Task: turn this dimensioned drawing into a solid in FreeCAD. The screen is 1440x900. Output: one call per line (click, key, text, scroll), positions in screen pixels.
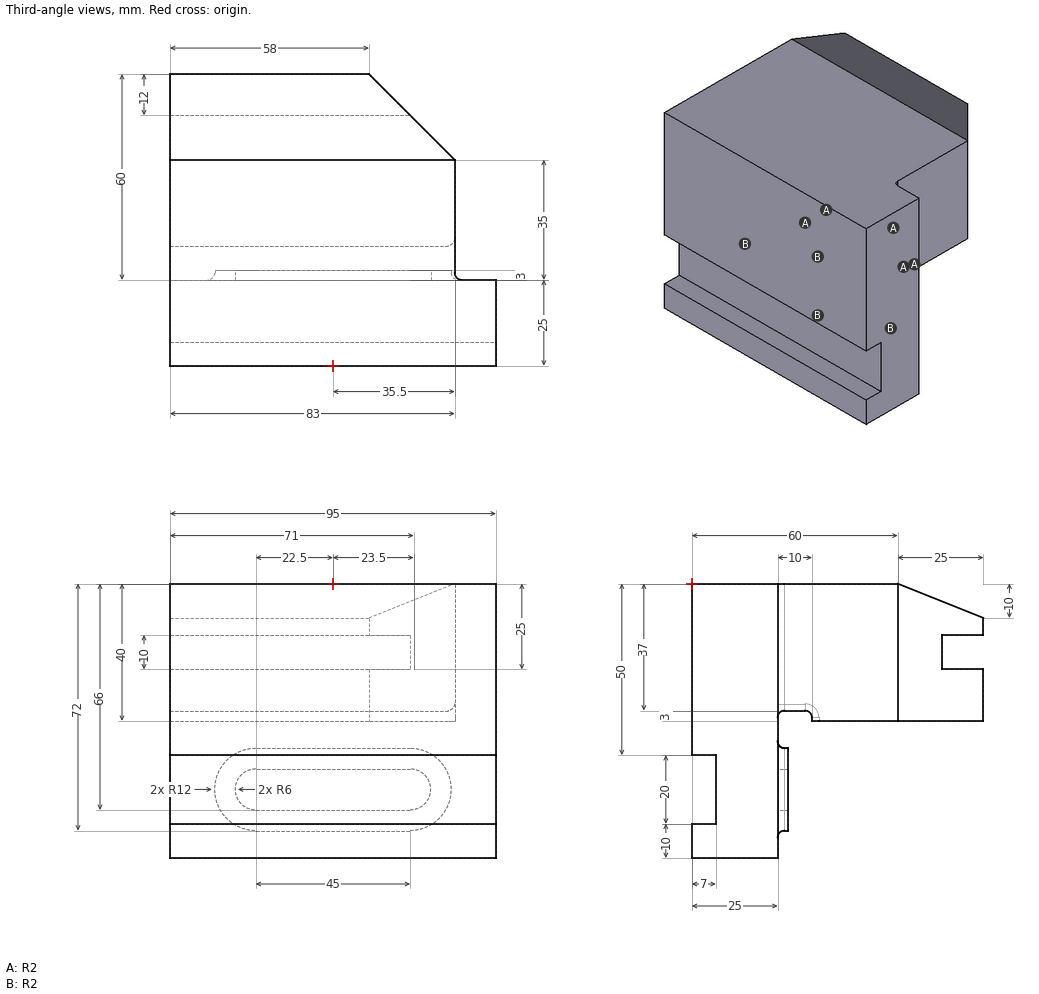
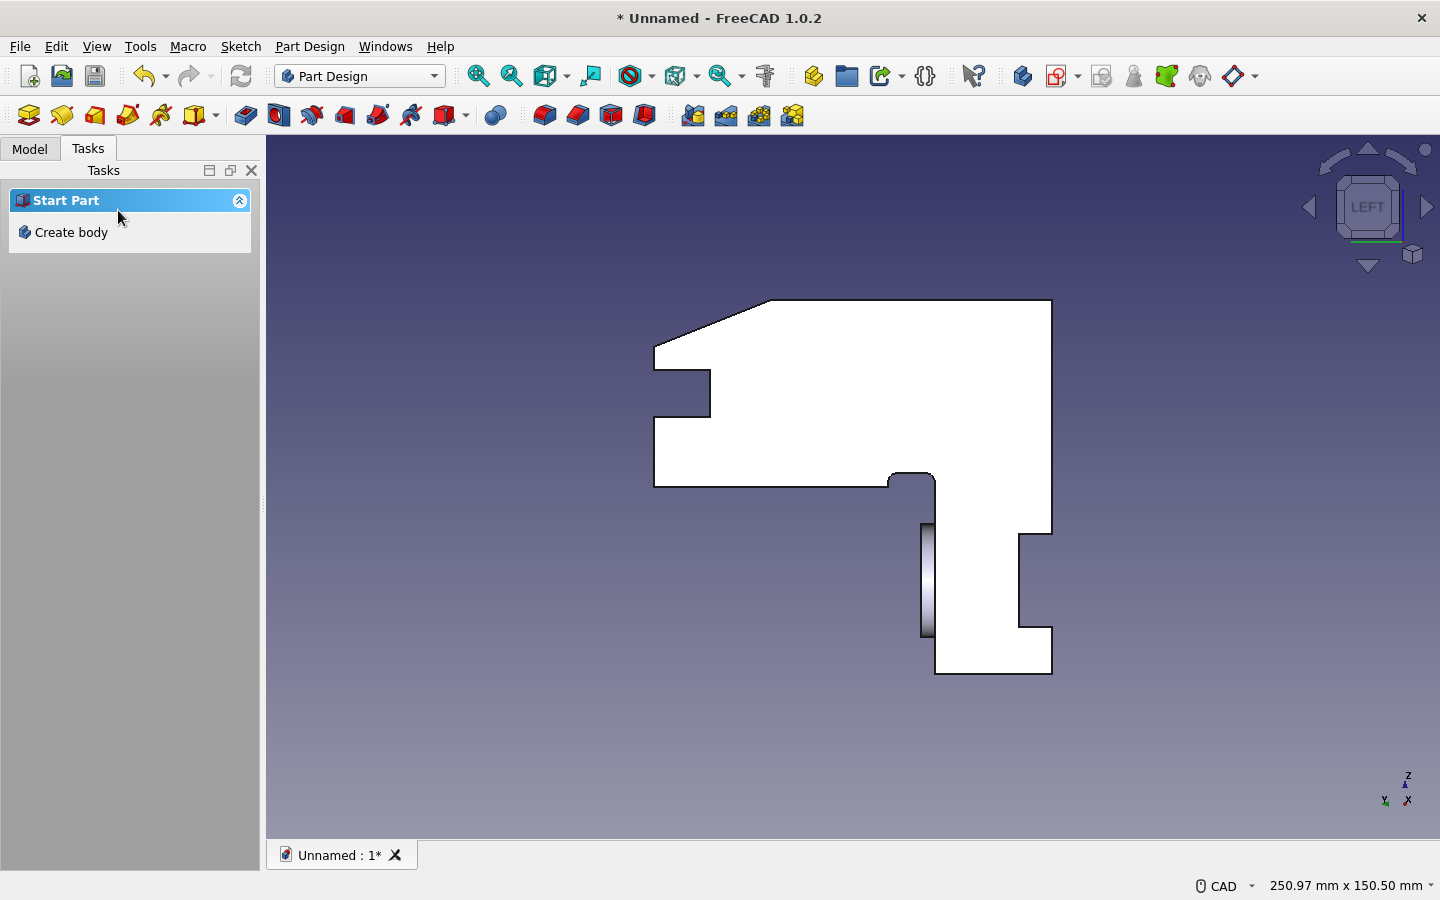
key(v)
key(3)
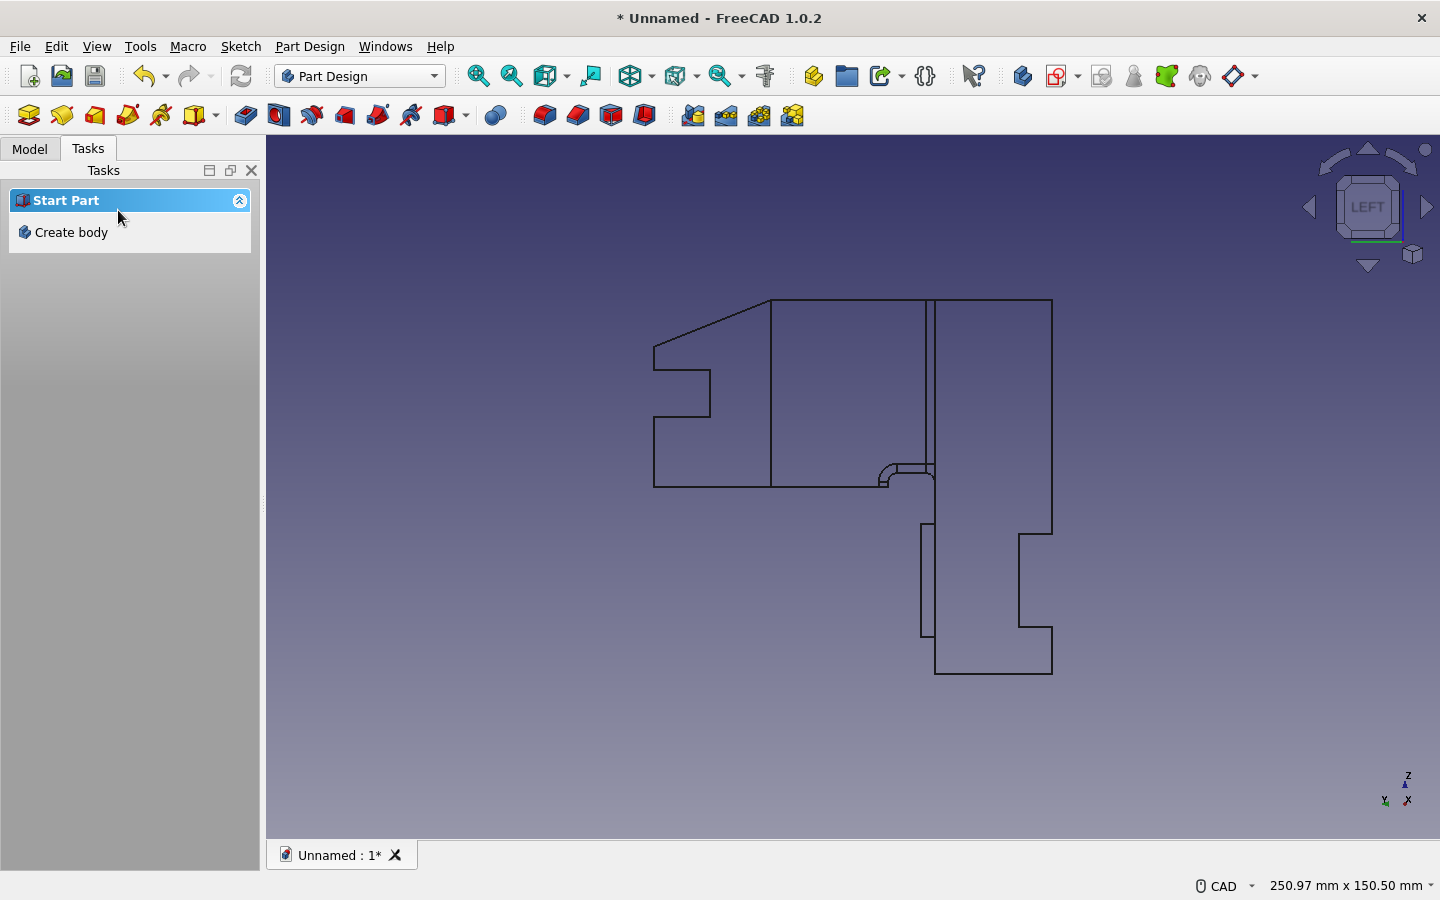
key(0)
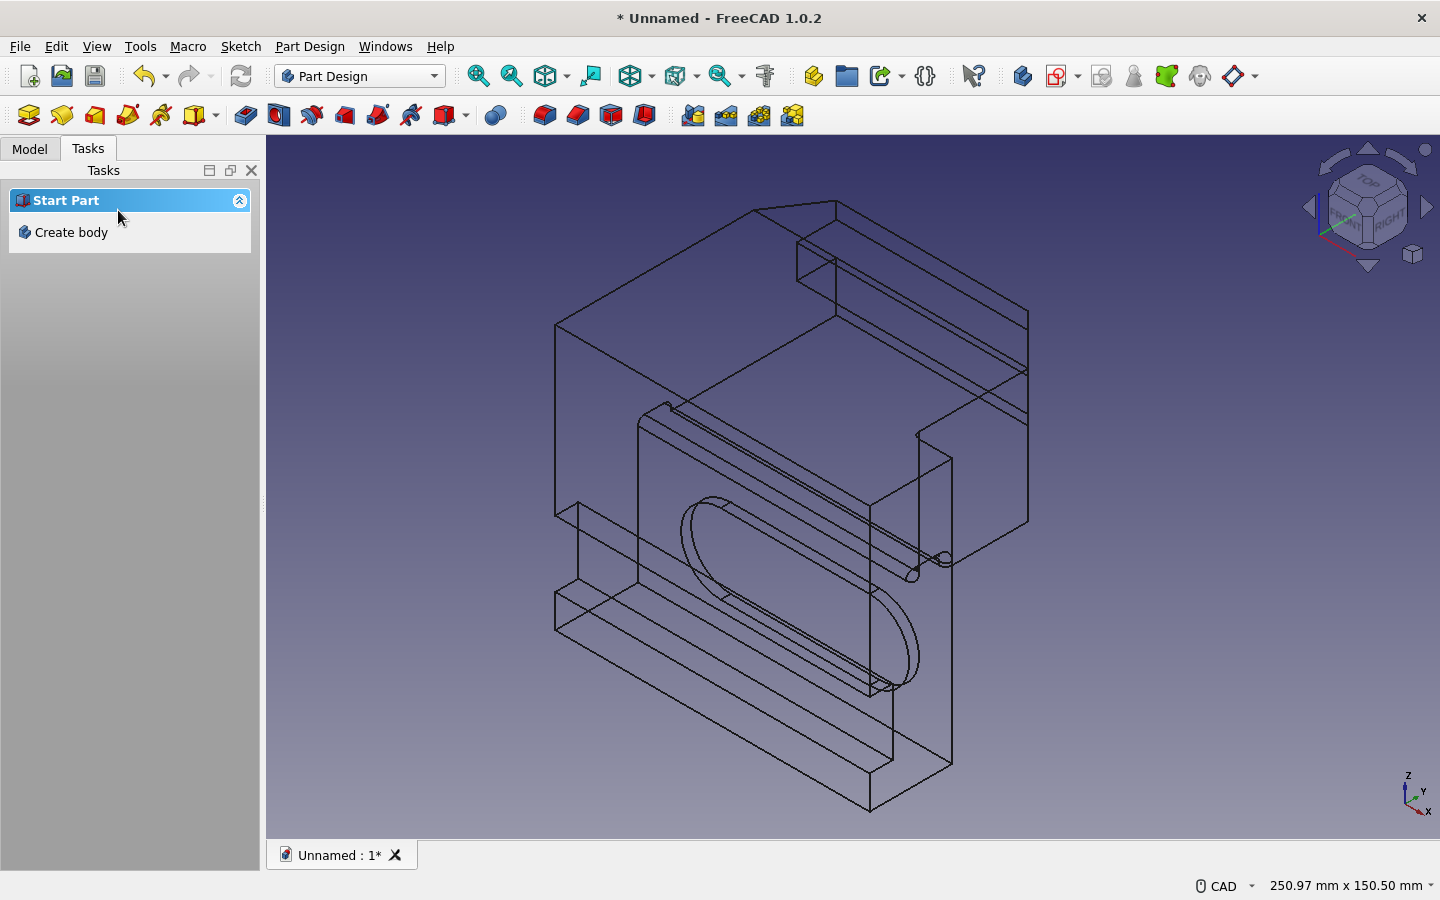
click(681, 530)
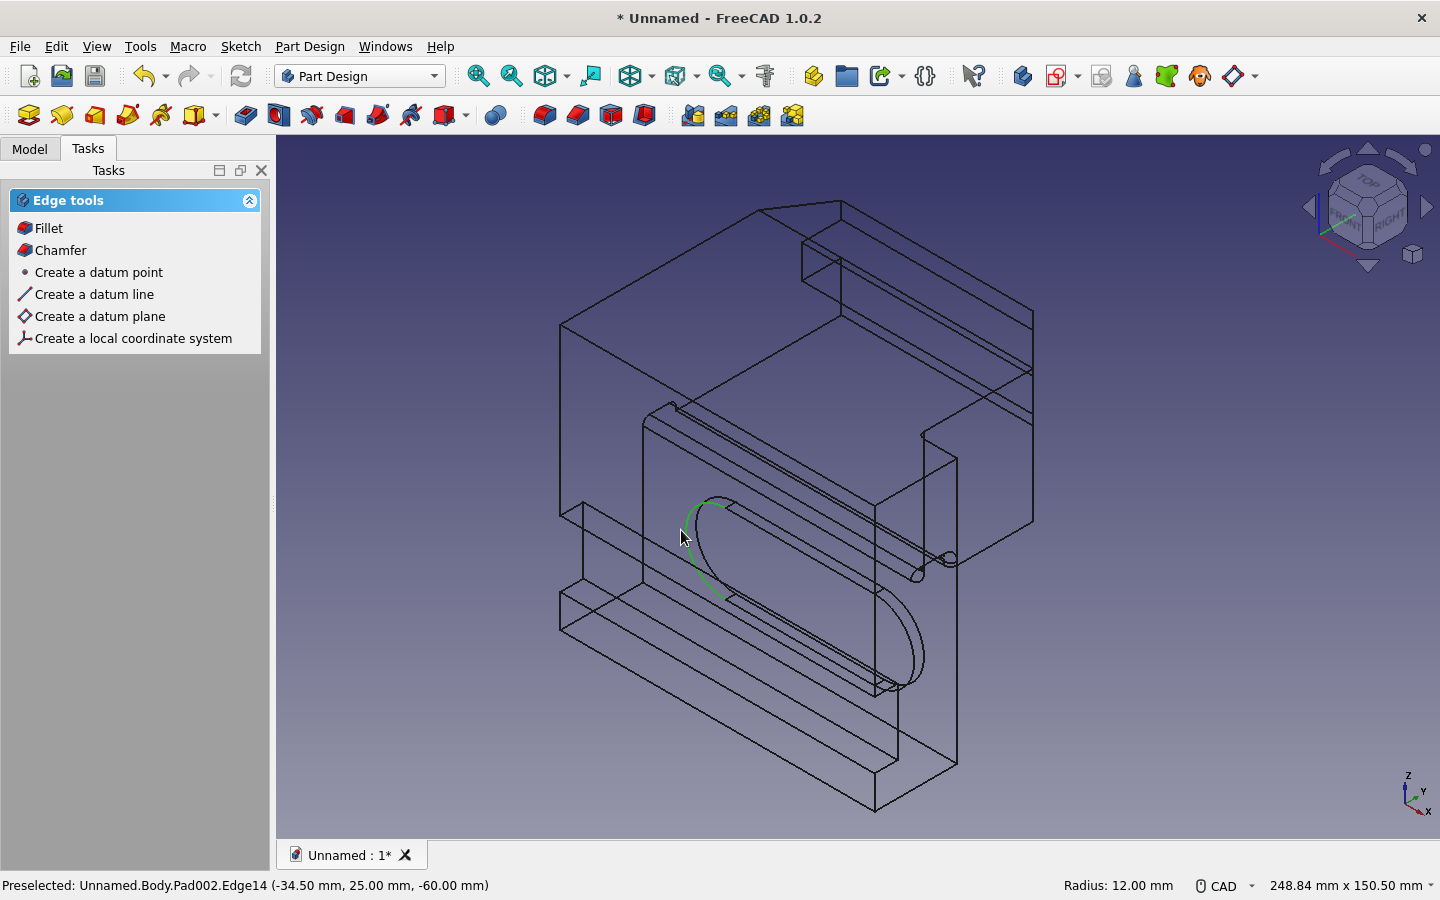
click(800, 550, ctrl)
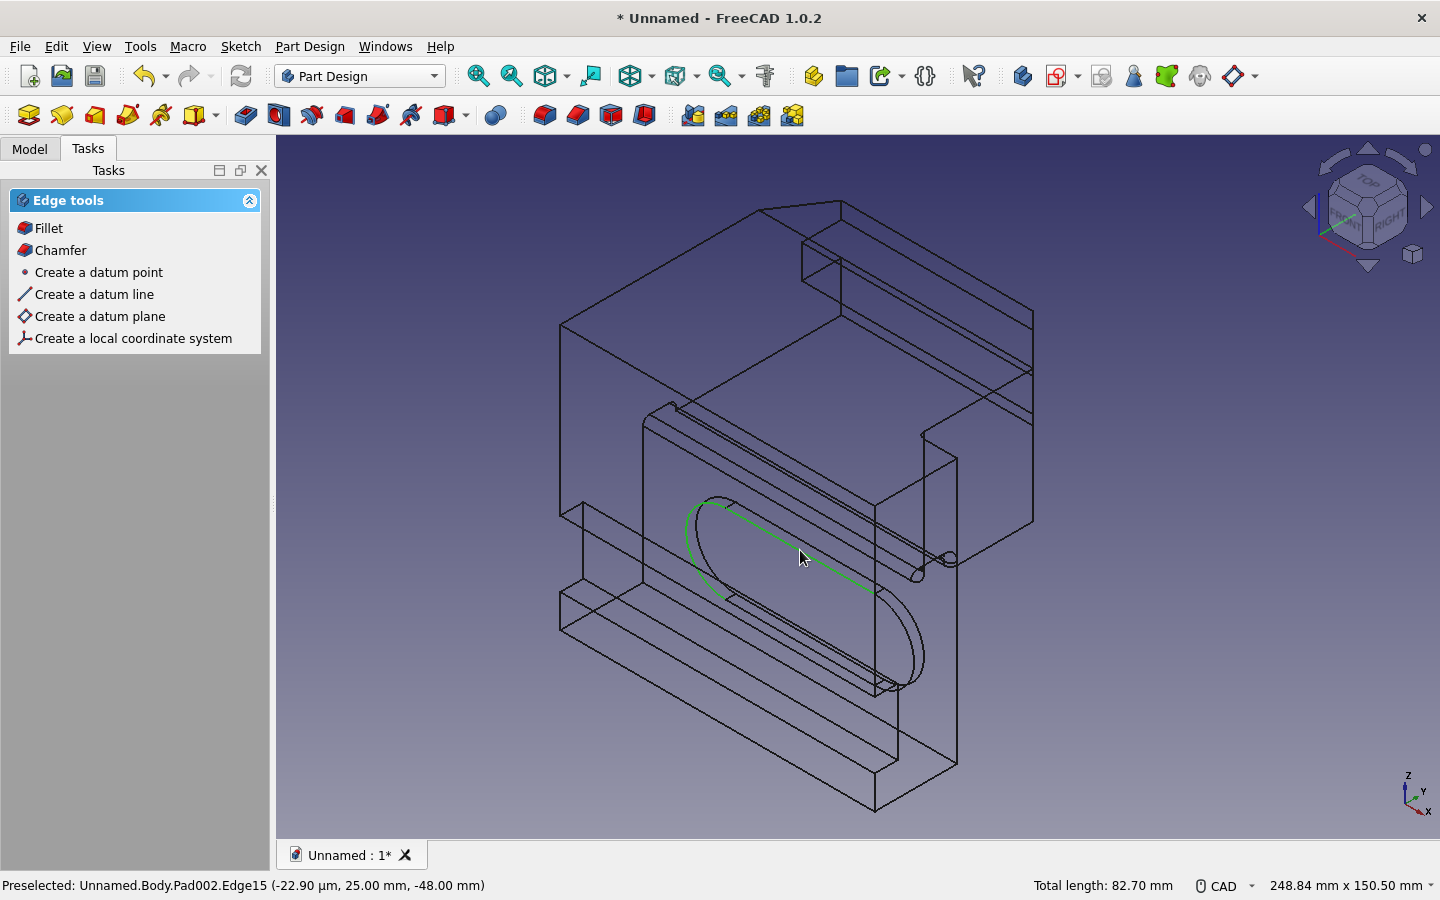
click(914, 662, ctrl)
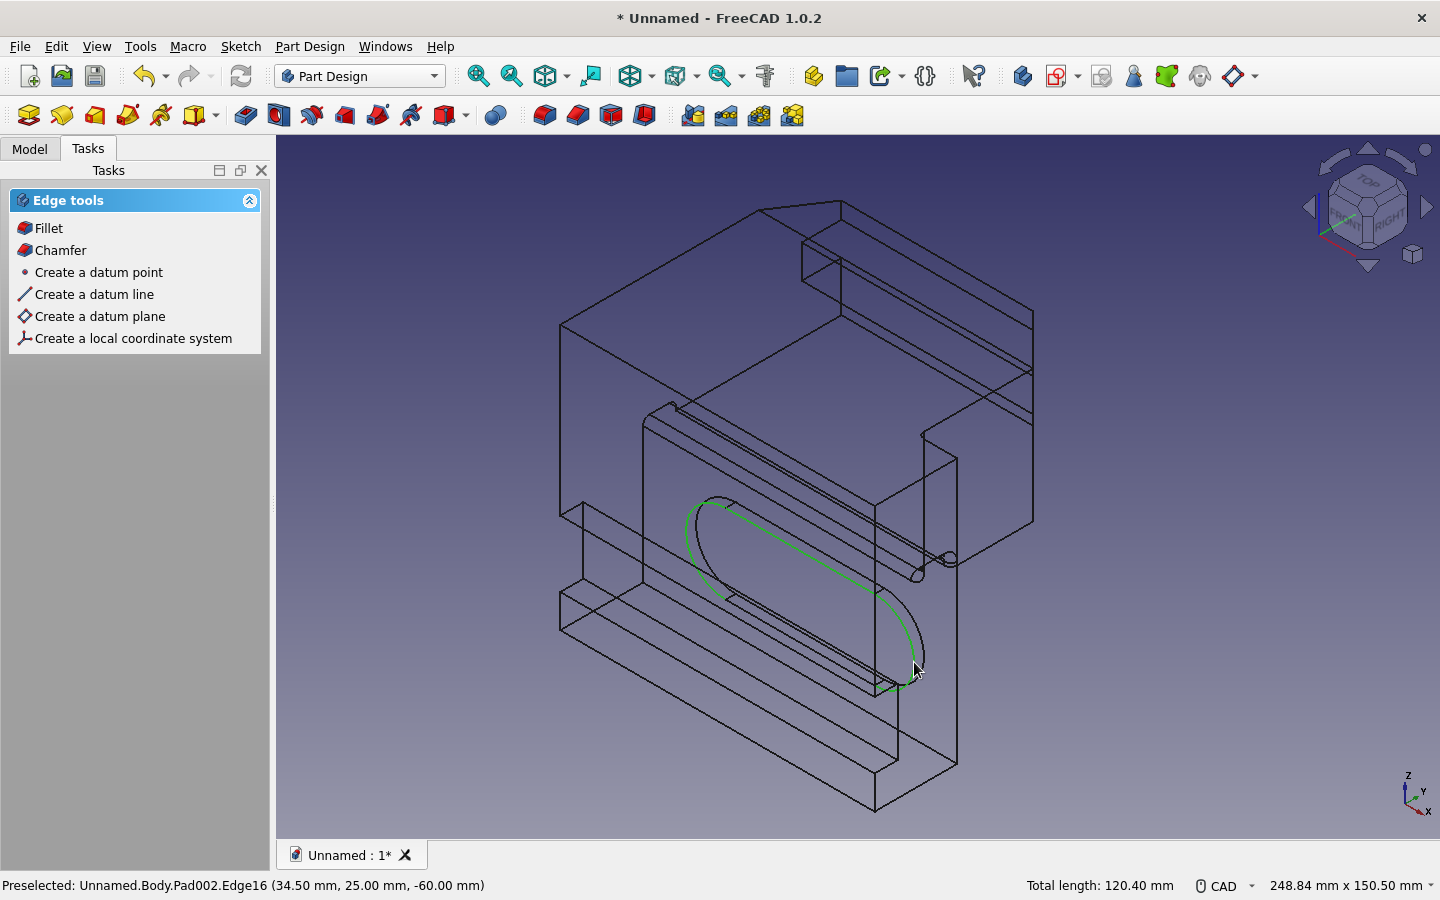
click(800, 642, ctrl)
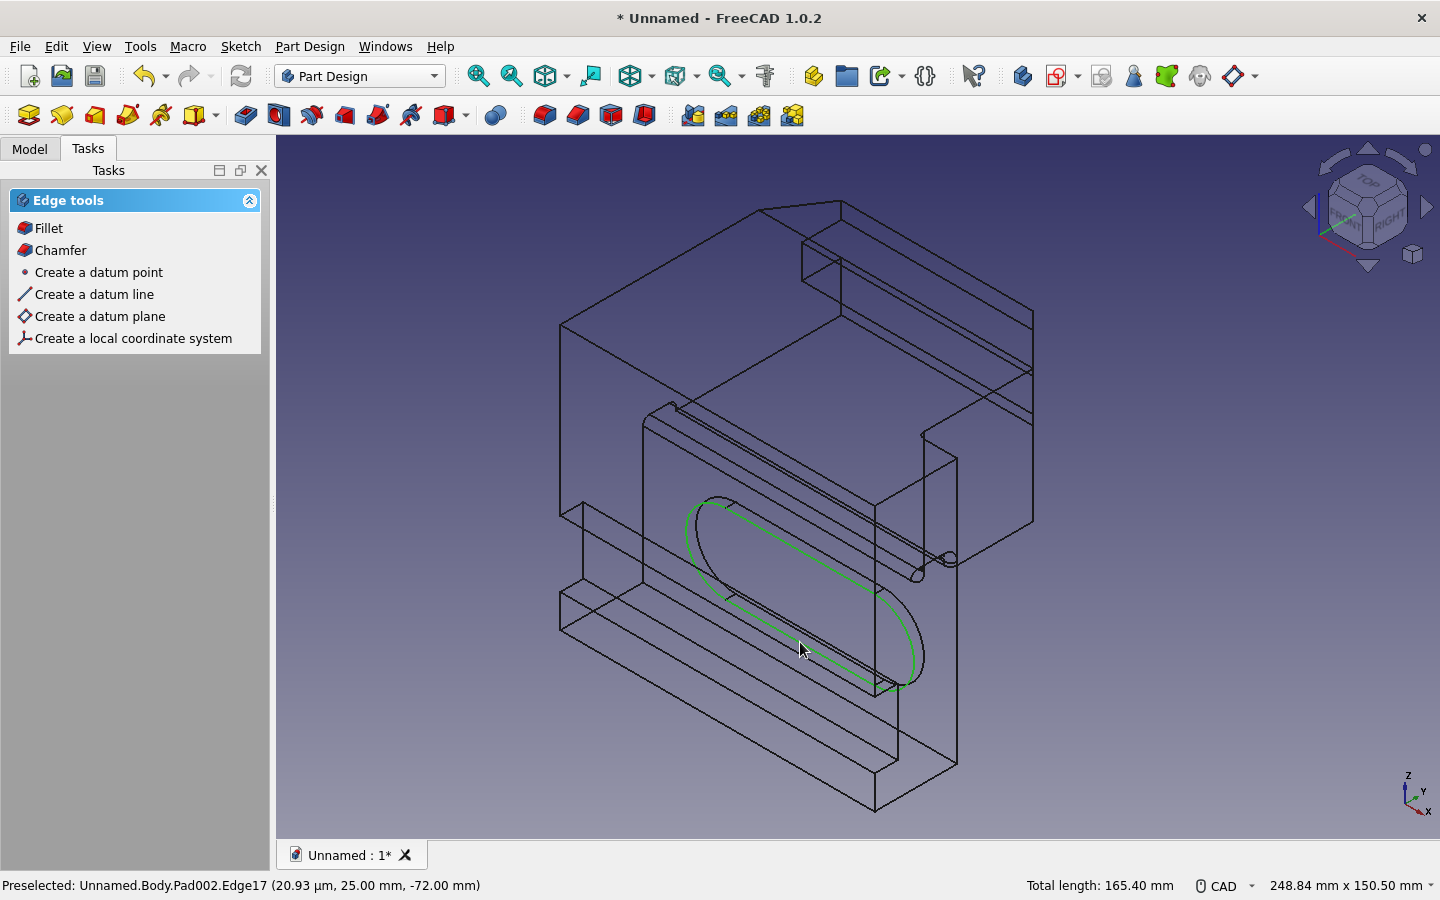
key(v)
key(1)